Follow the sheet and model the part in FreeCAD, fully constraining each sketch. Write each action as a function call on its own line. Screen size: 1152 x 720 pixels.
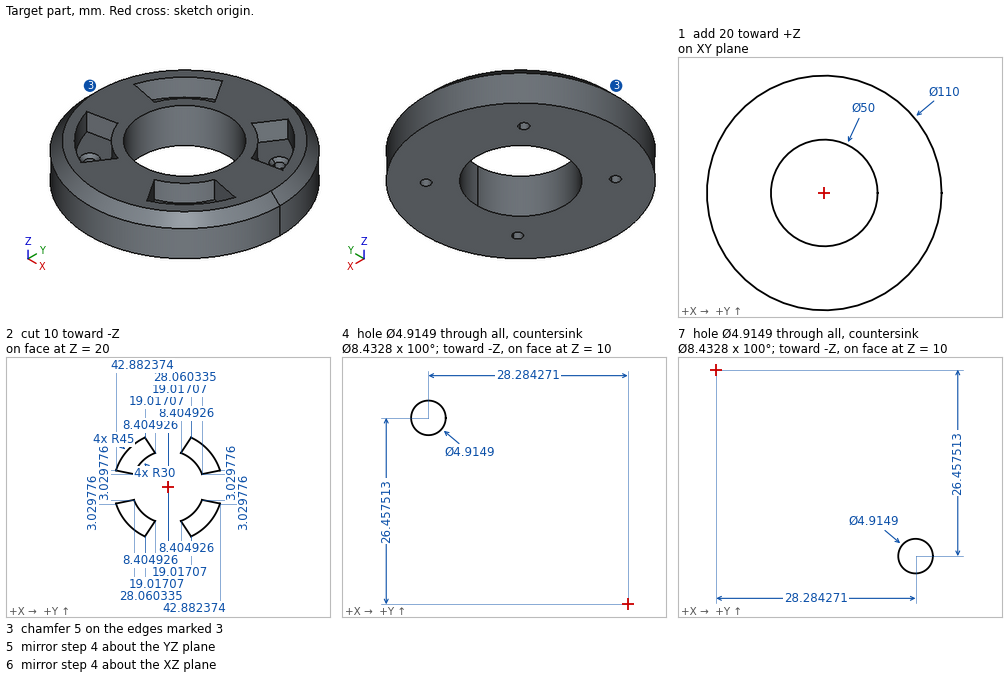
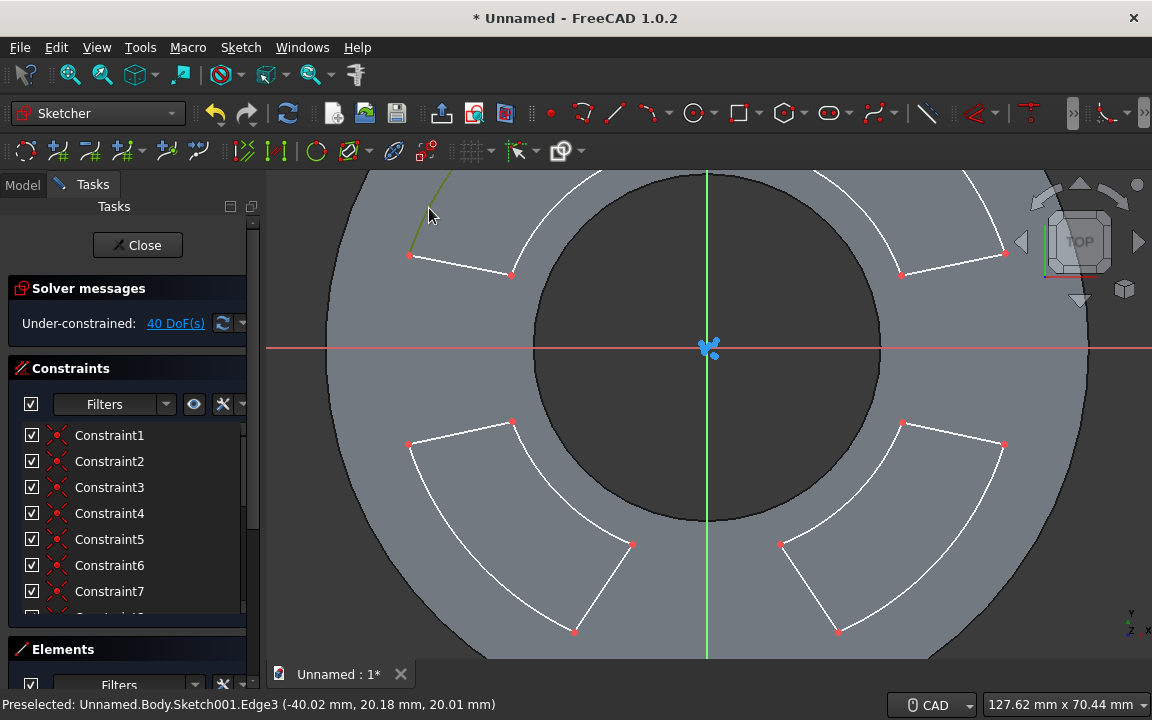
click(537, 229)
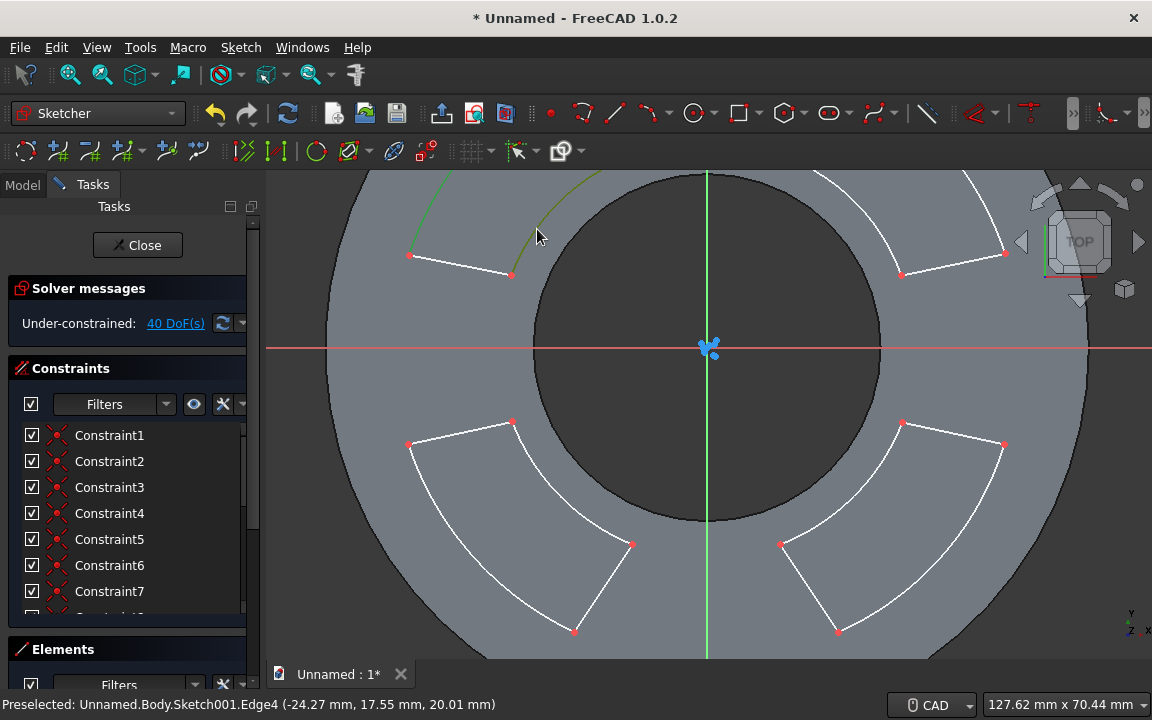
click(1030, 114)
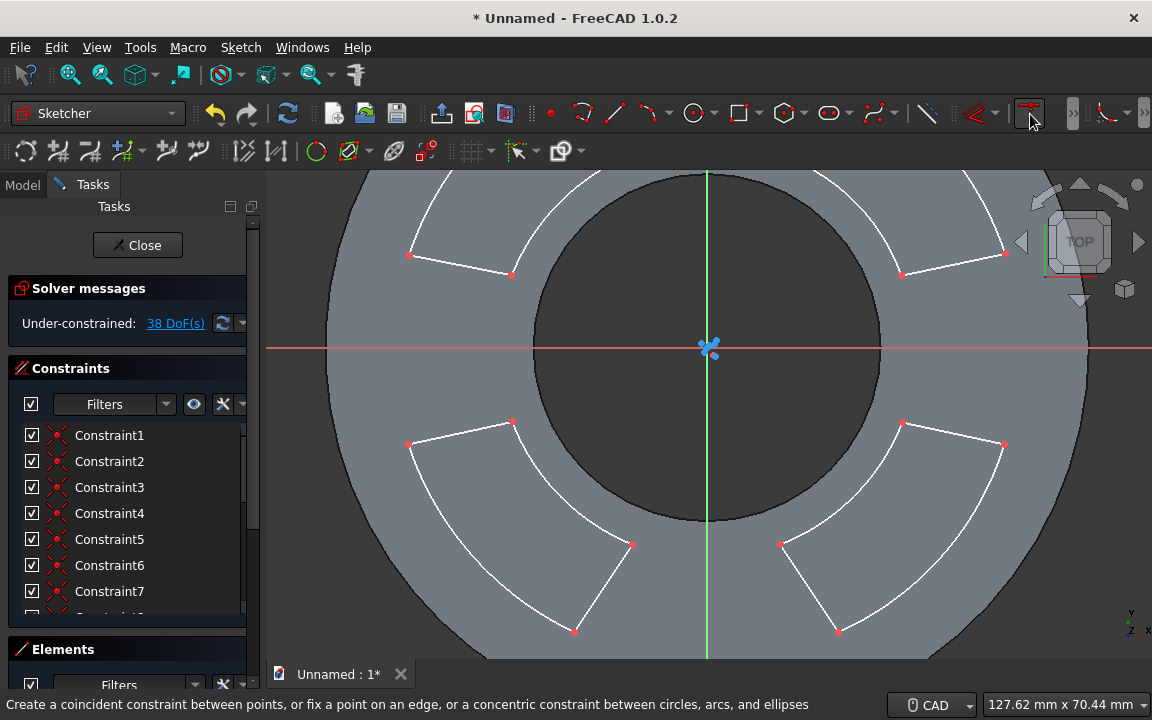
click(429, 208)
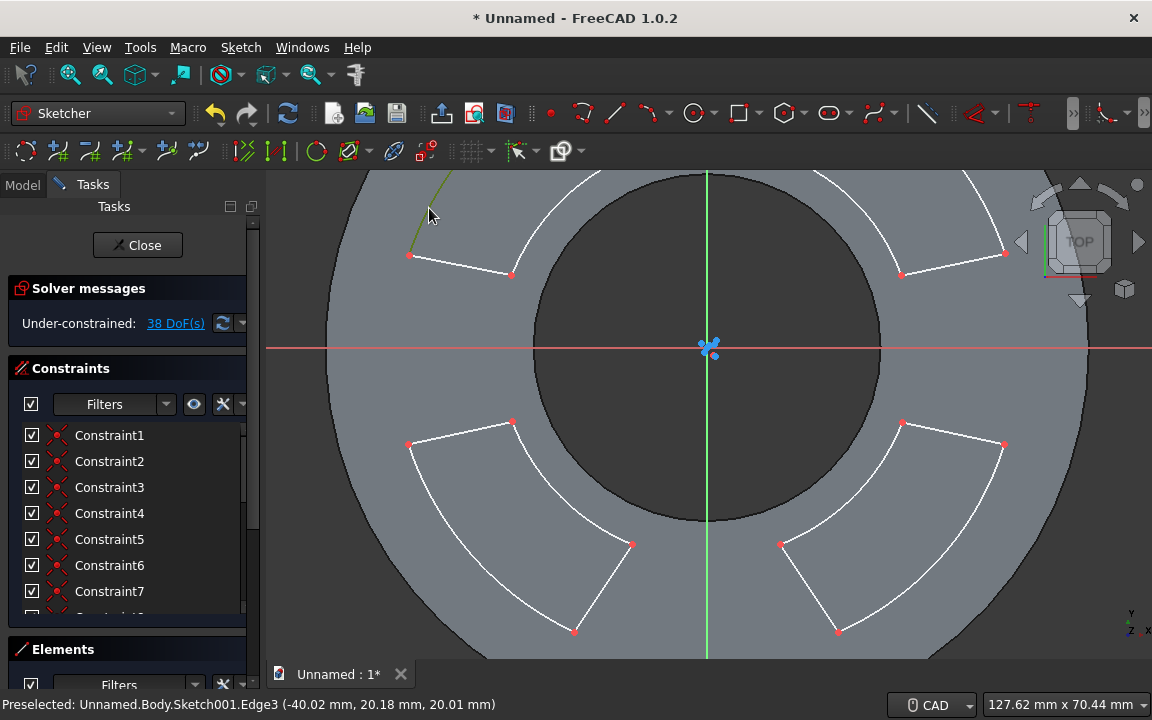
click(985, 207)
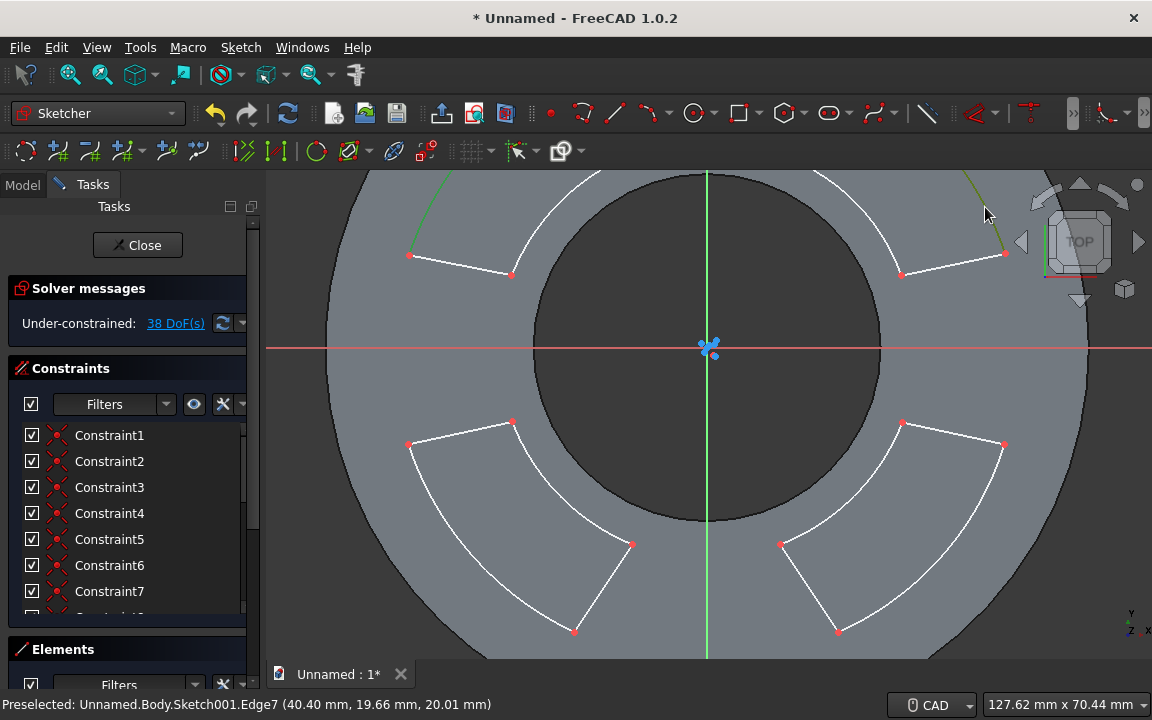
click(1030, 114)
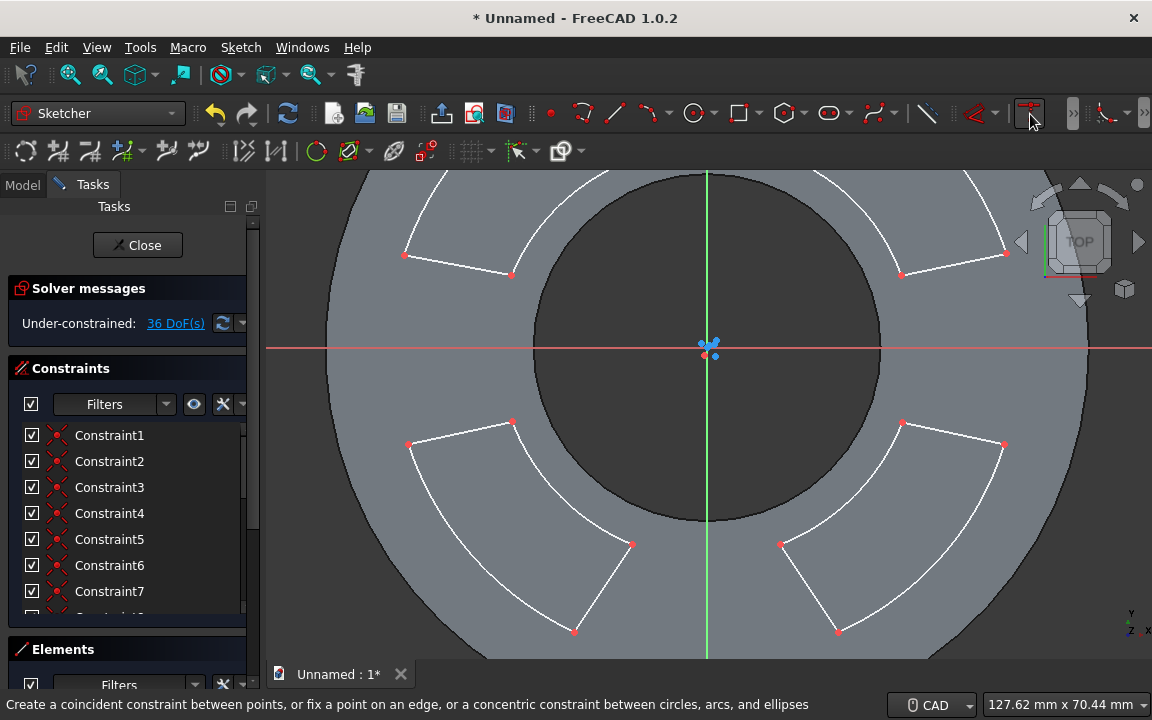
click(425, 207)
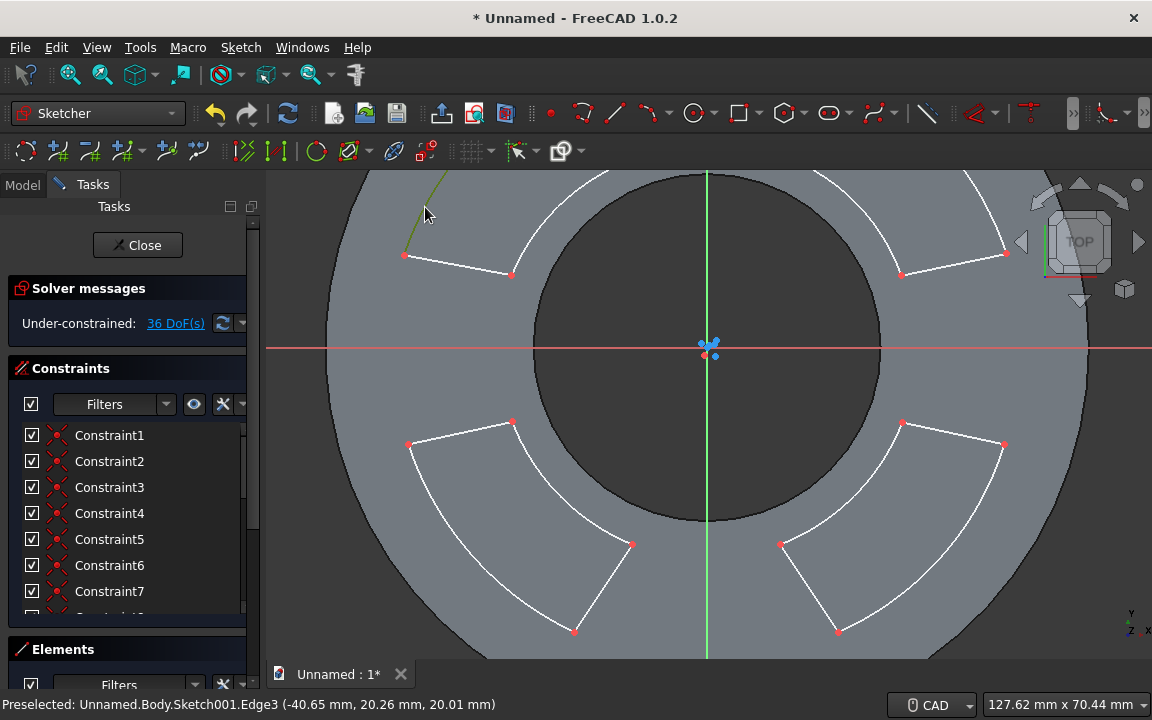
click(877, 229)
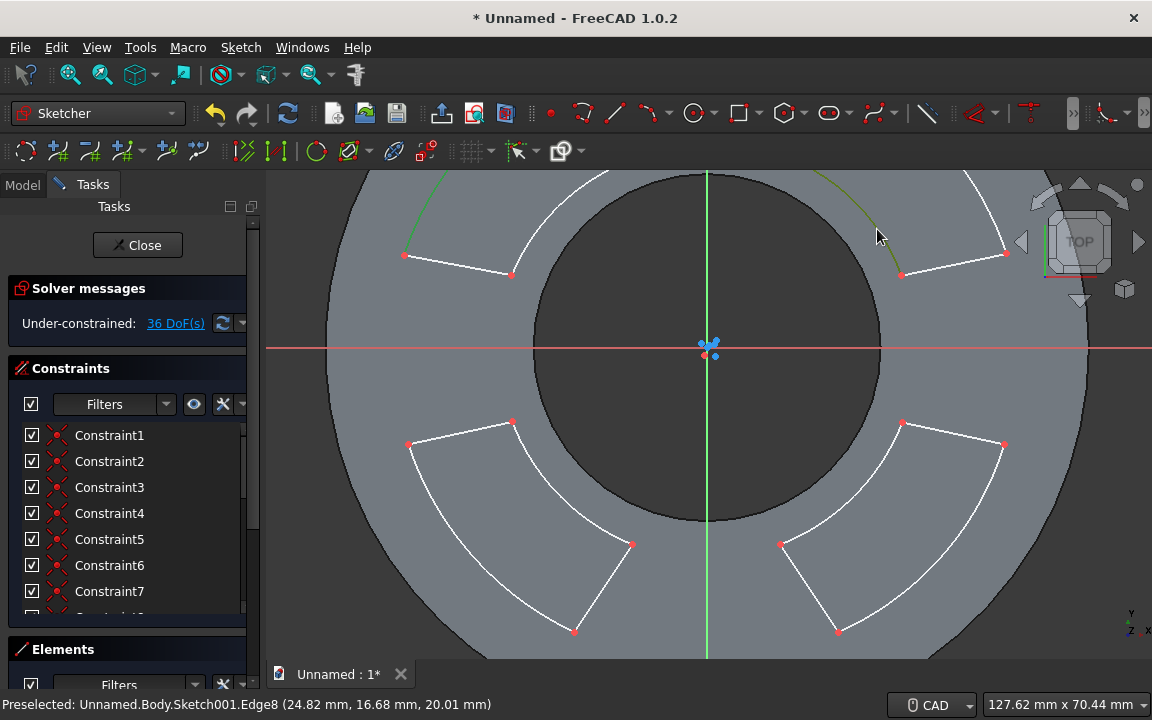
click(1030, 114)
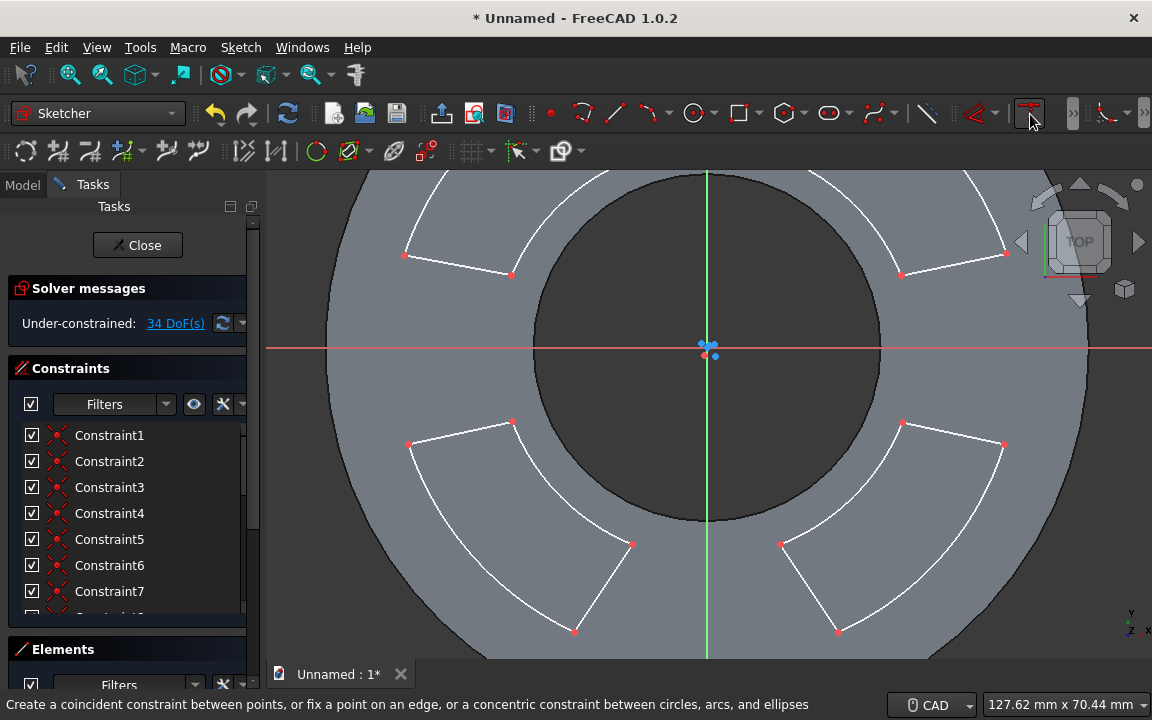
click(425, 207)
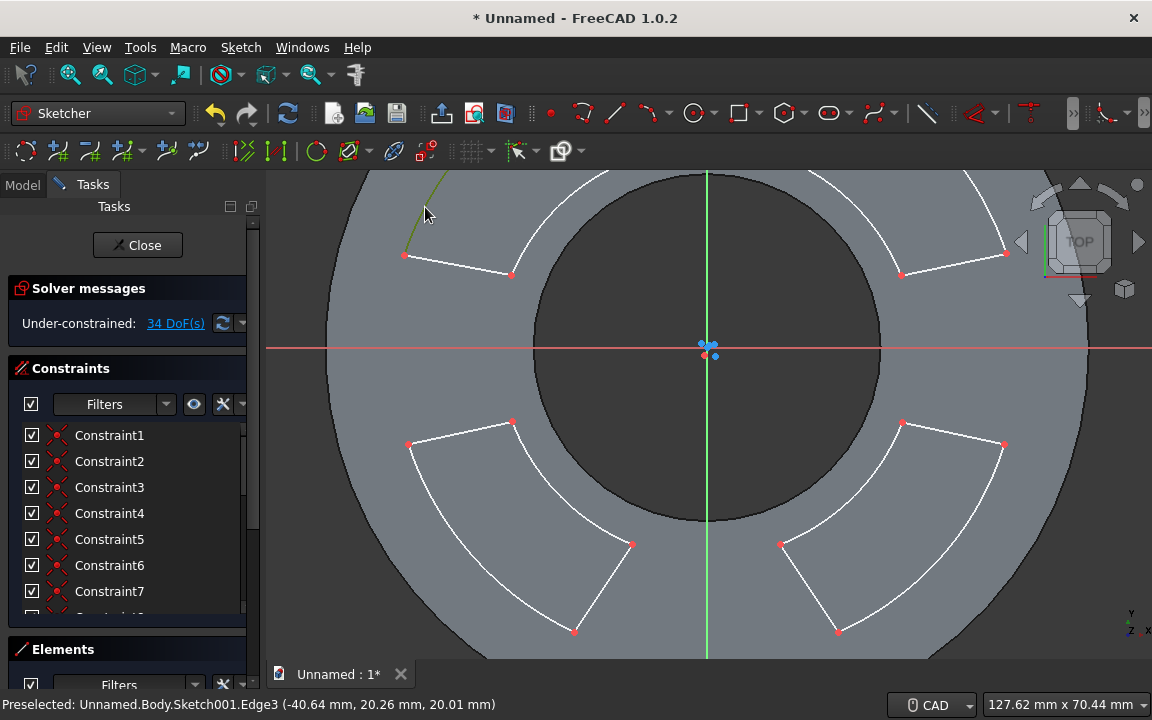
click(904, 592)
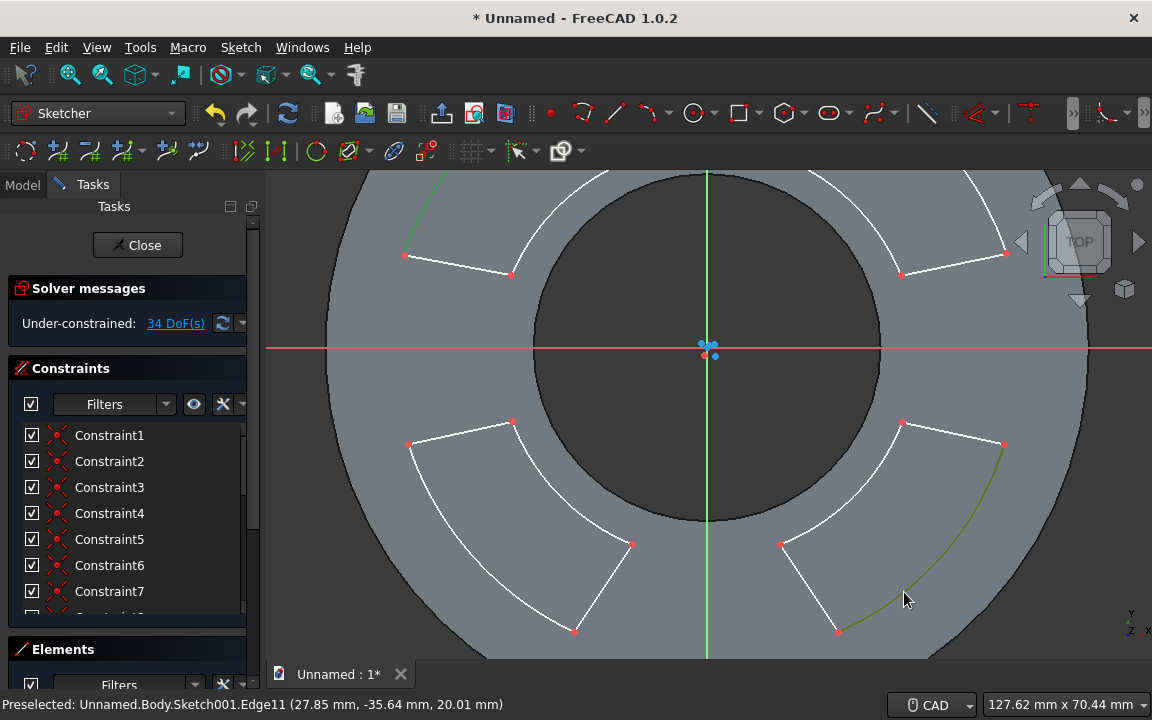
click(1030, 114)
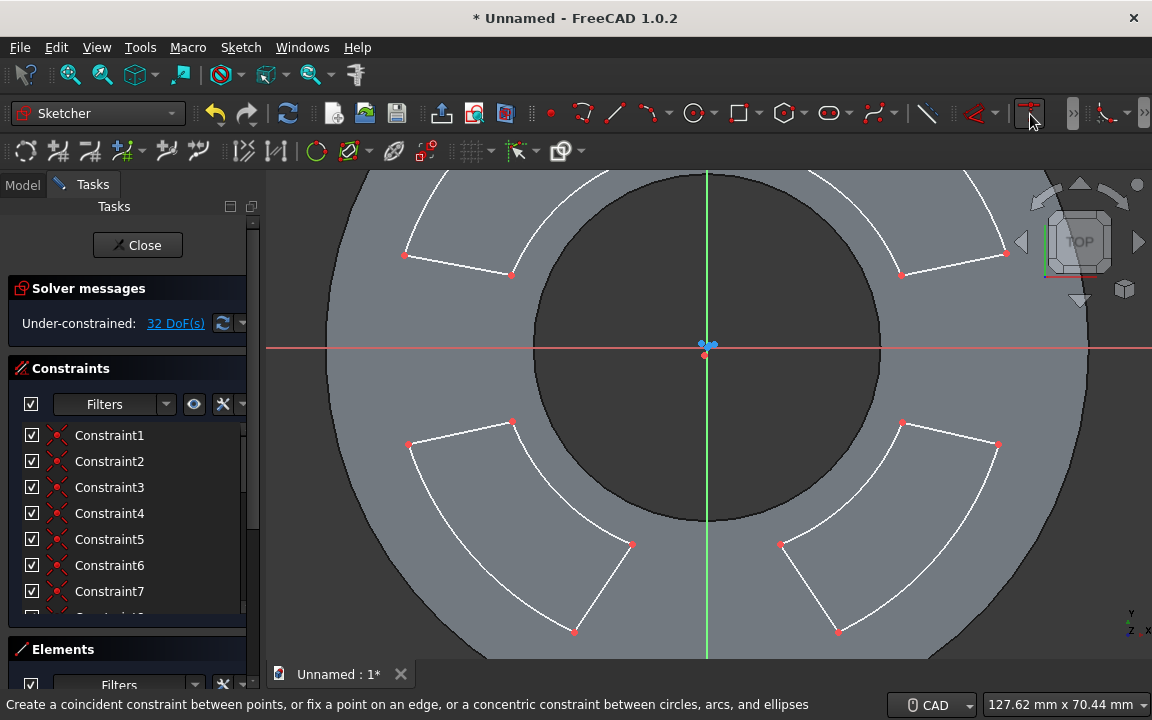
click(425, 207)